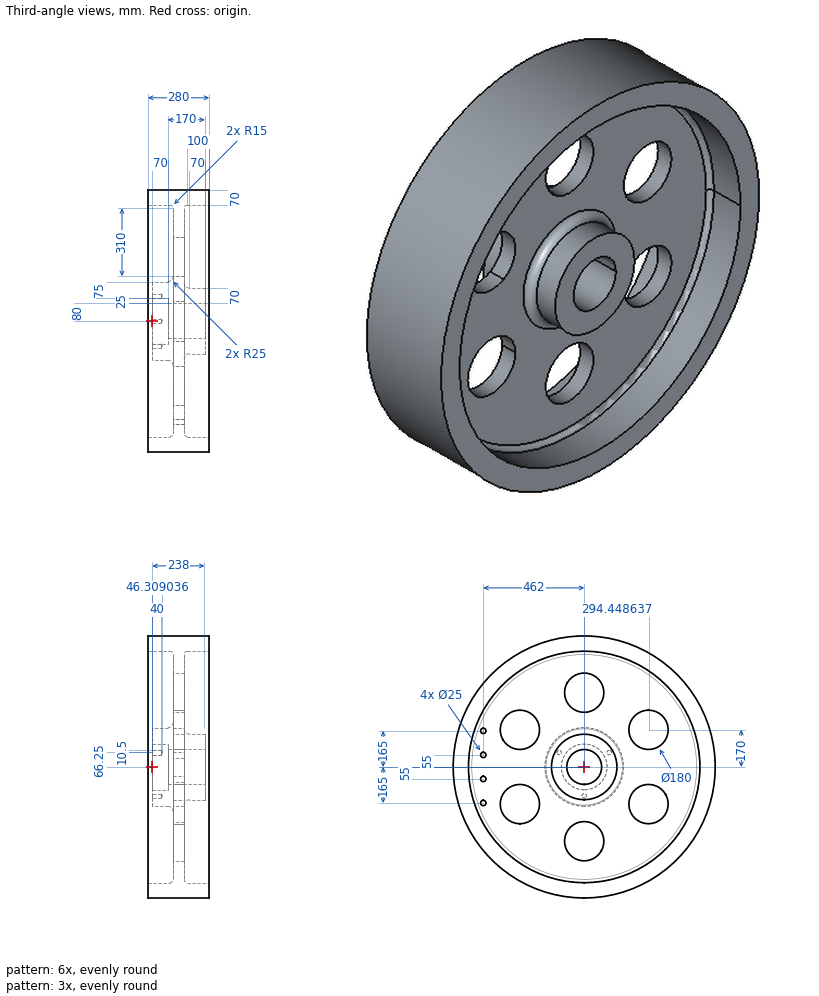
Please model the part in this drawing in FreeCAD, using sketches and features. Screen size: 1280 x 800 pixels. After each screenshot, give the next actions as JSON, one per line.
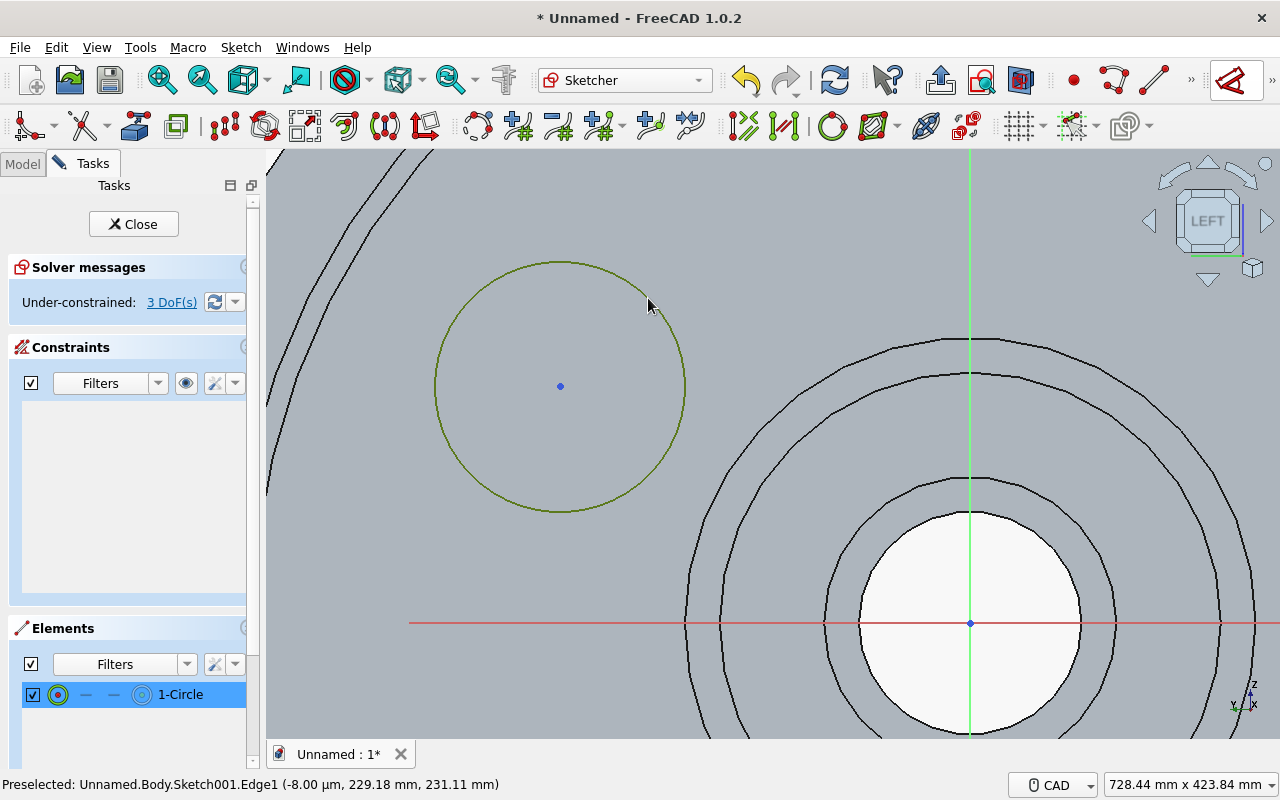
{"action": "key", "text": "k o"}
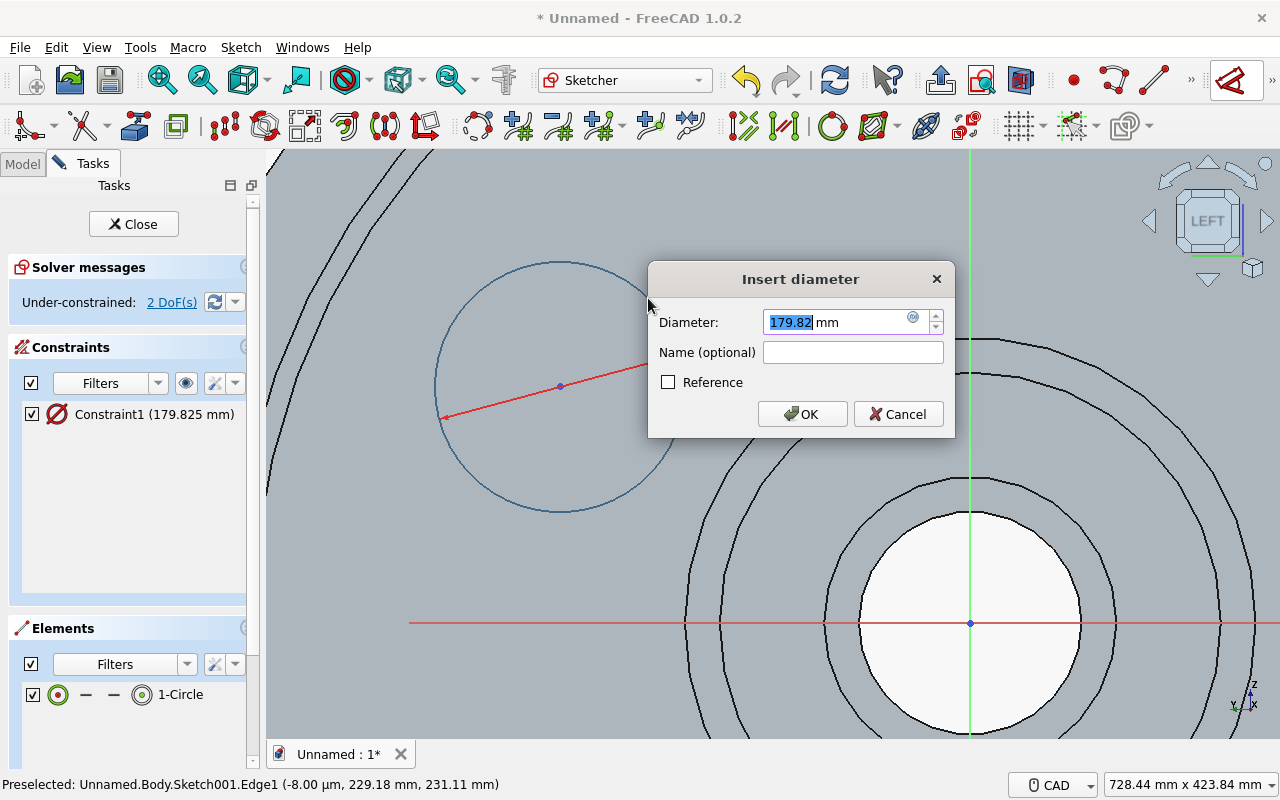
{"action": "type", "text": "180"}
{"action": "key", "text": "Return"}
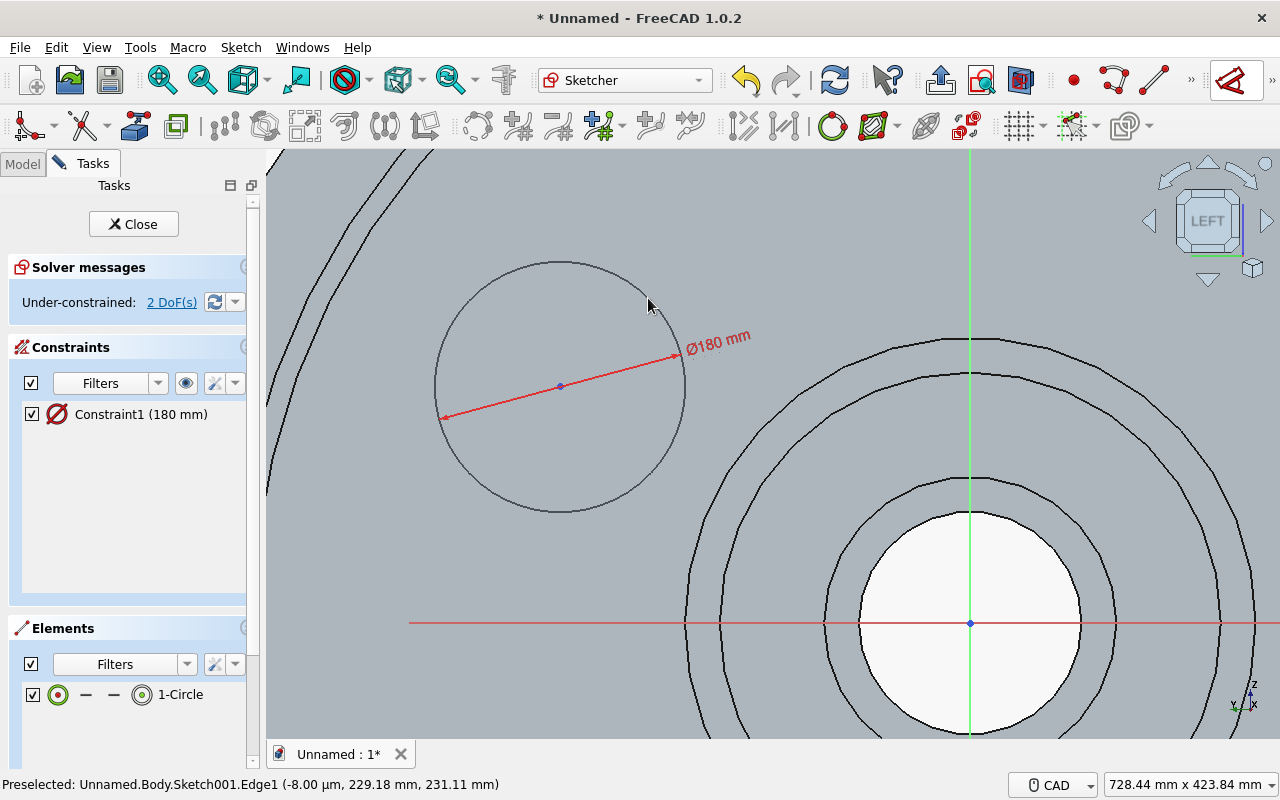
{"action": "left_click", "coordinate": [560, 387]}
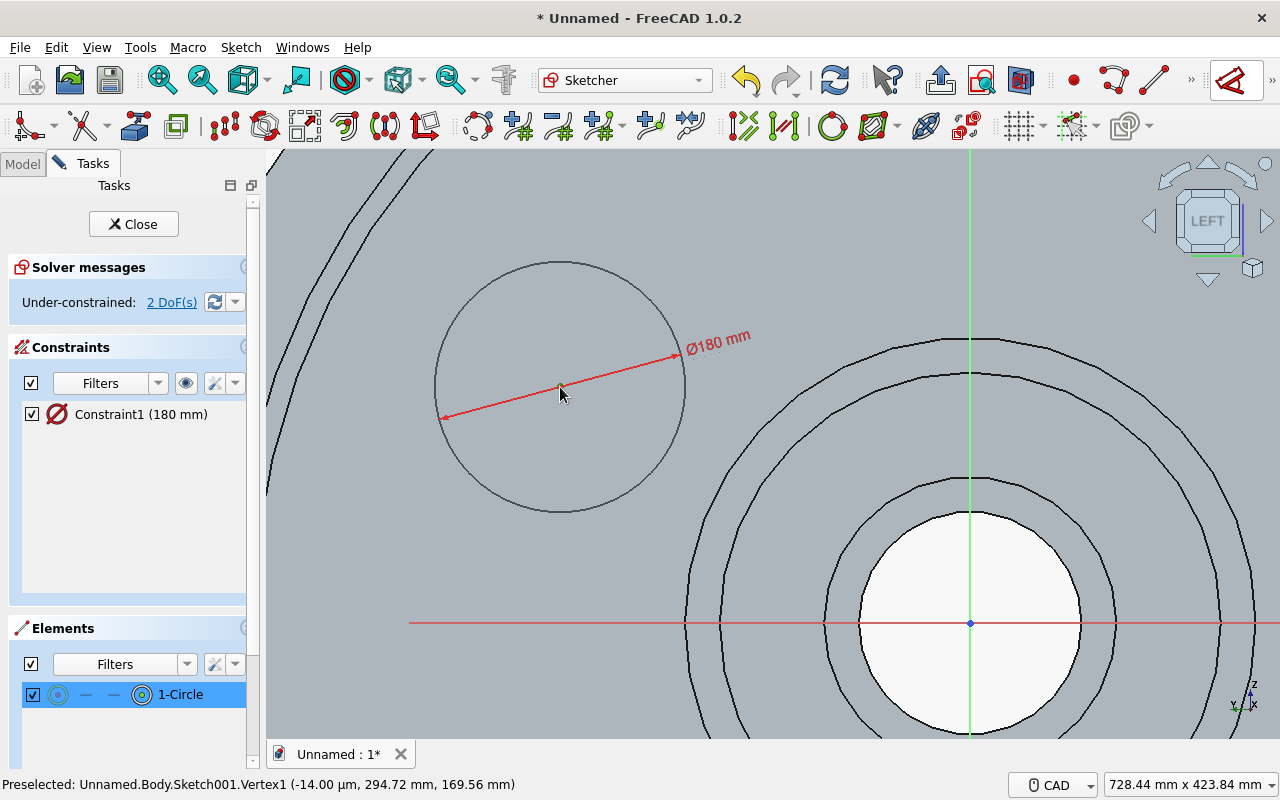
{"action": "key", "text": "i"}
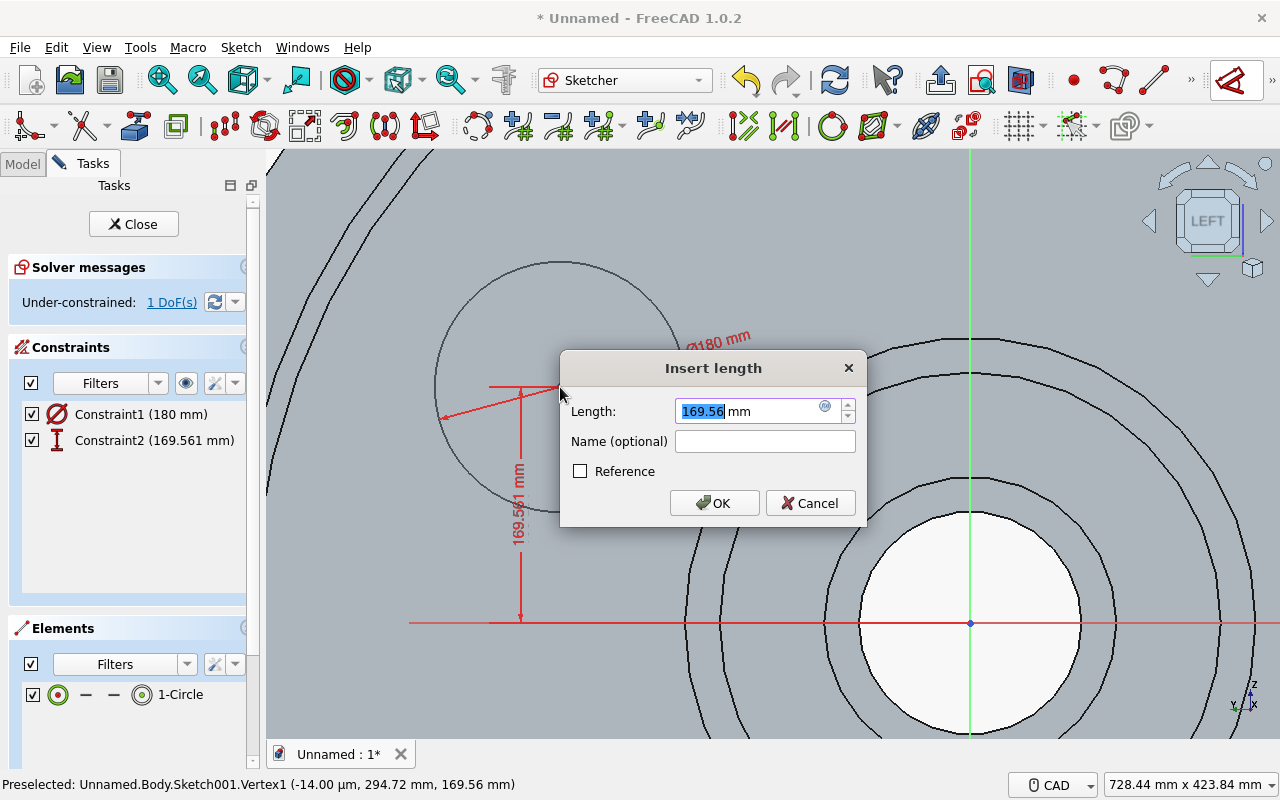
{"action": "type", "text": "170"}
{"action": "key", "text": "Return"}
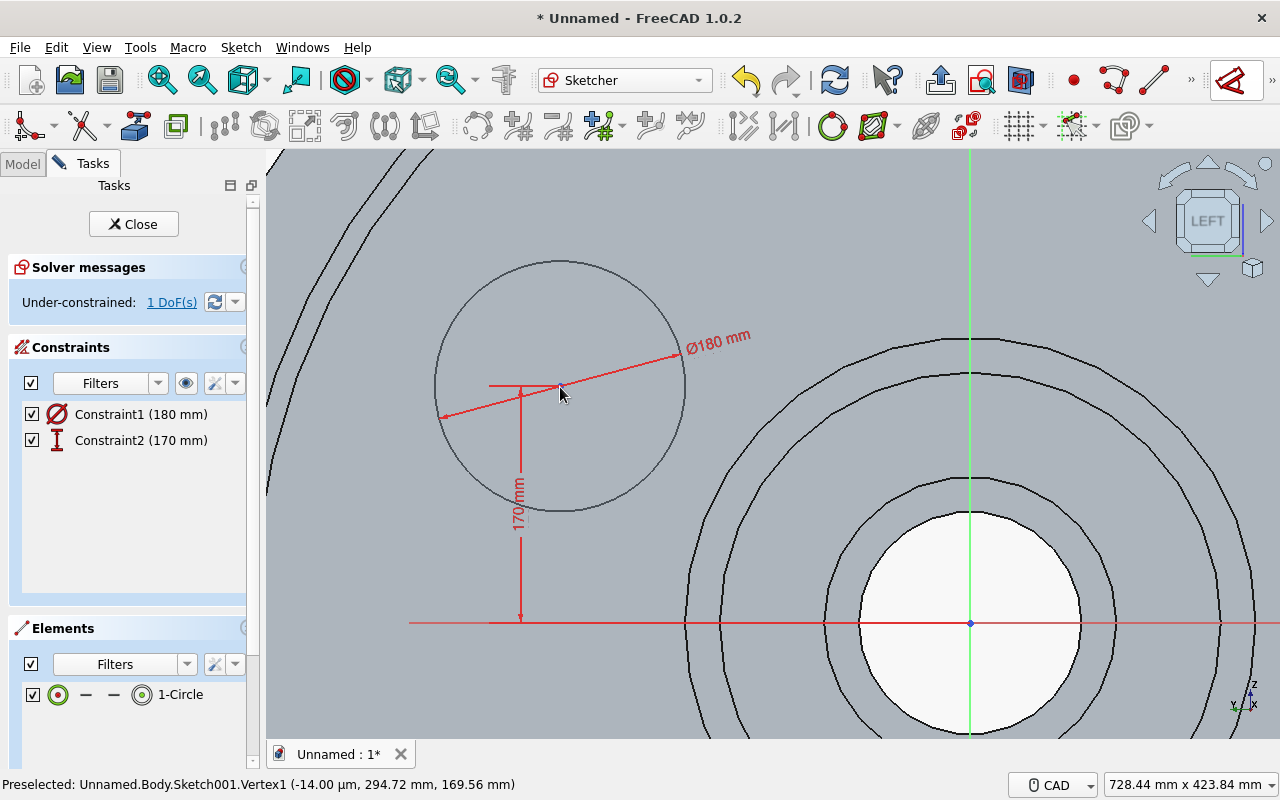
{"action": "left_click", "coordinate": [560, 386]}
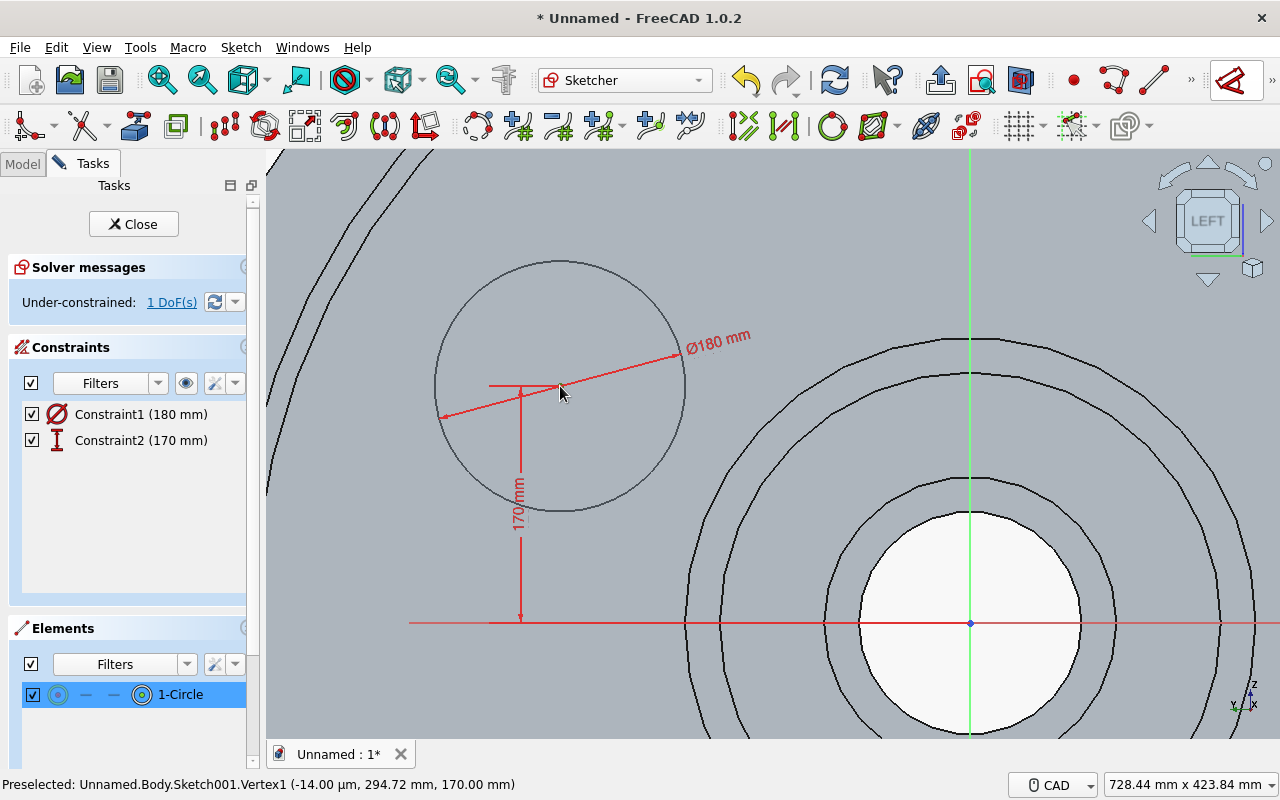
{"action": "left_click", "coordinate": [1258, 80]}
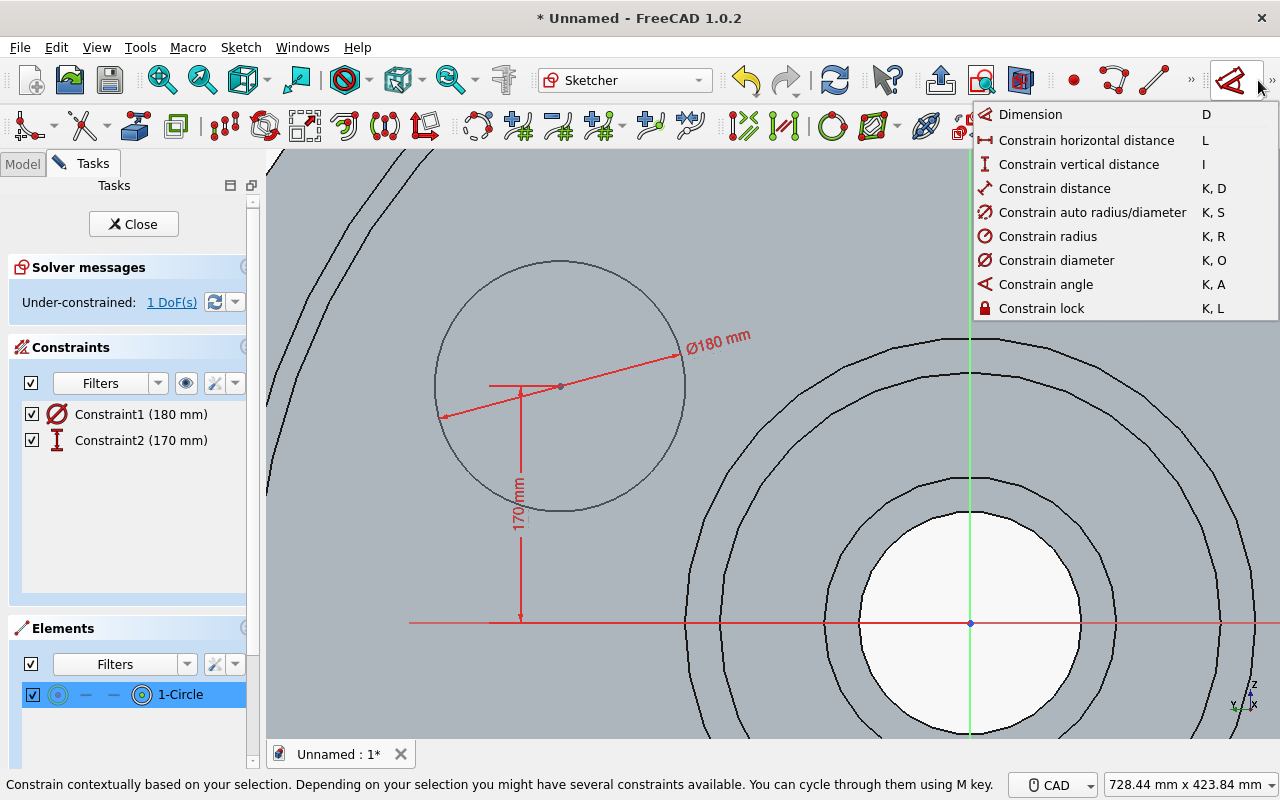
{"action": "left_click", "coordinate": [1126, 140]}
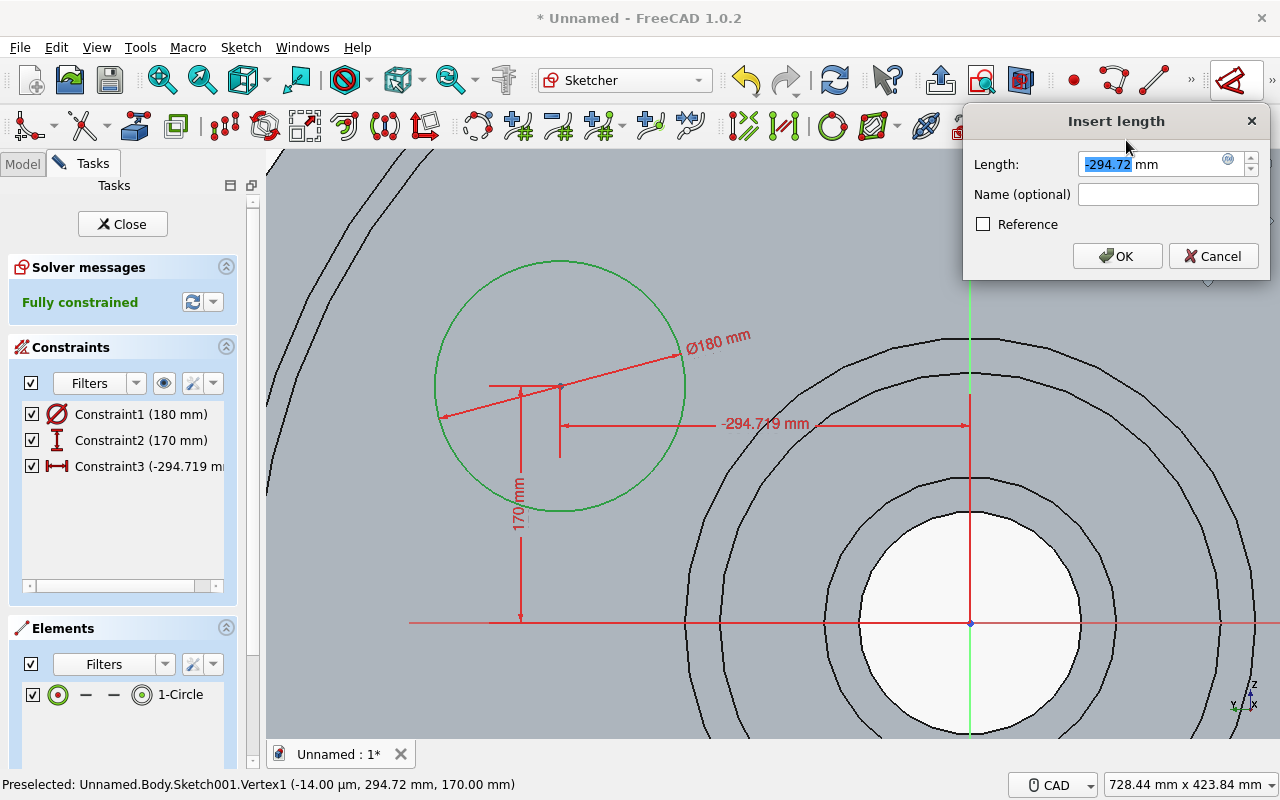
{"action": "type", "text": "-294.448637"}
{"action": "key", "text": "Return"}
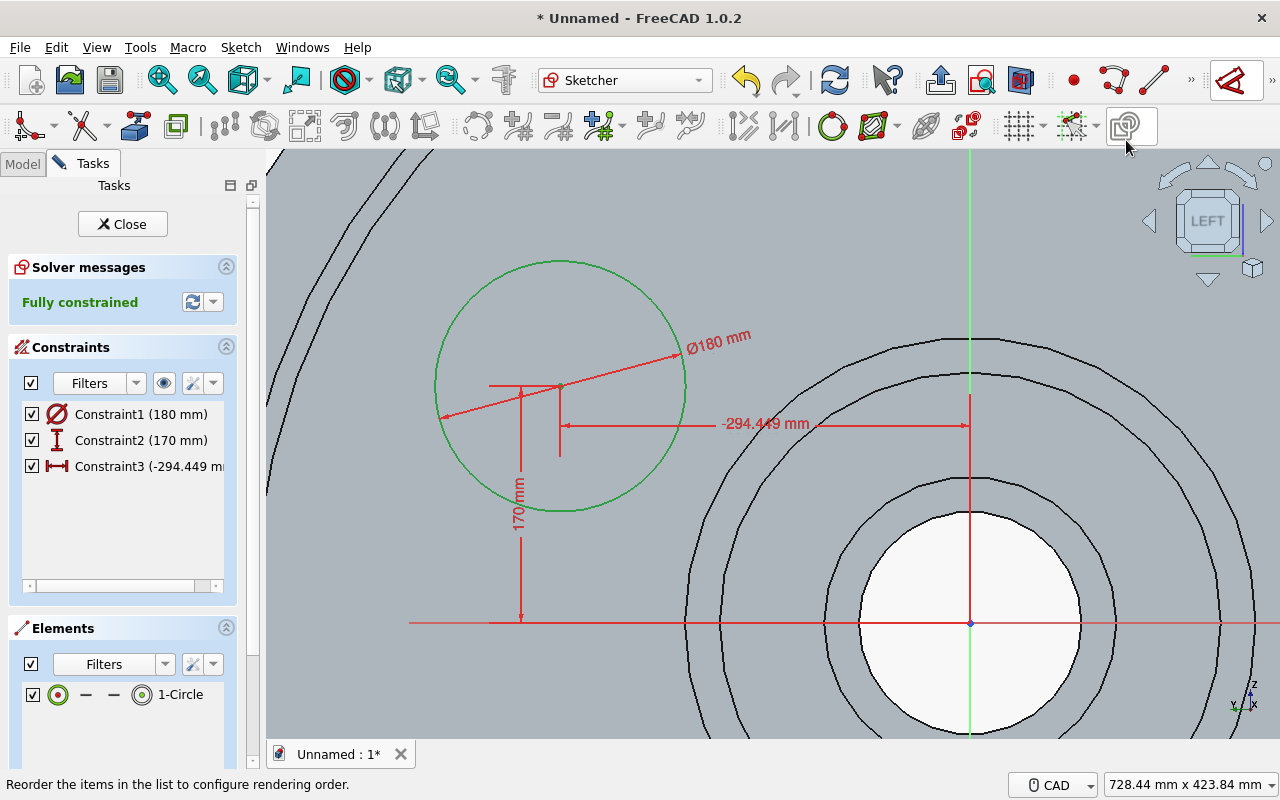
{"action": "left_click", "coordinate": [123, 224]}